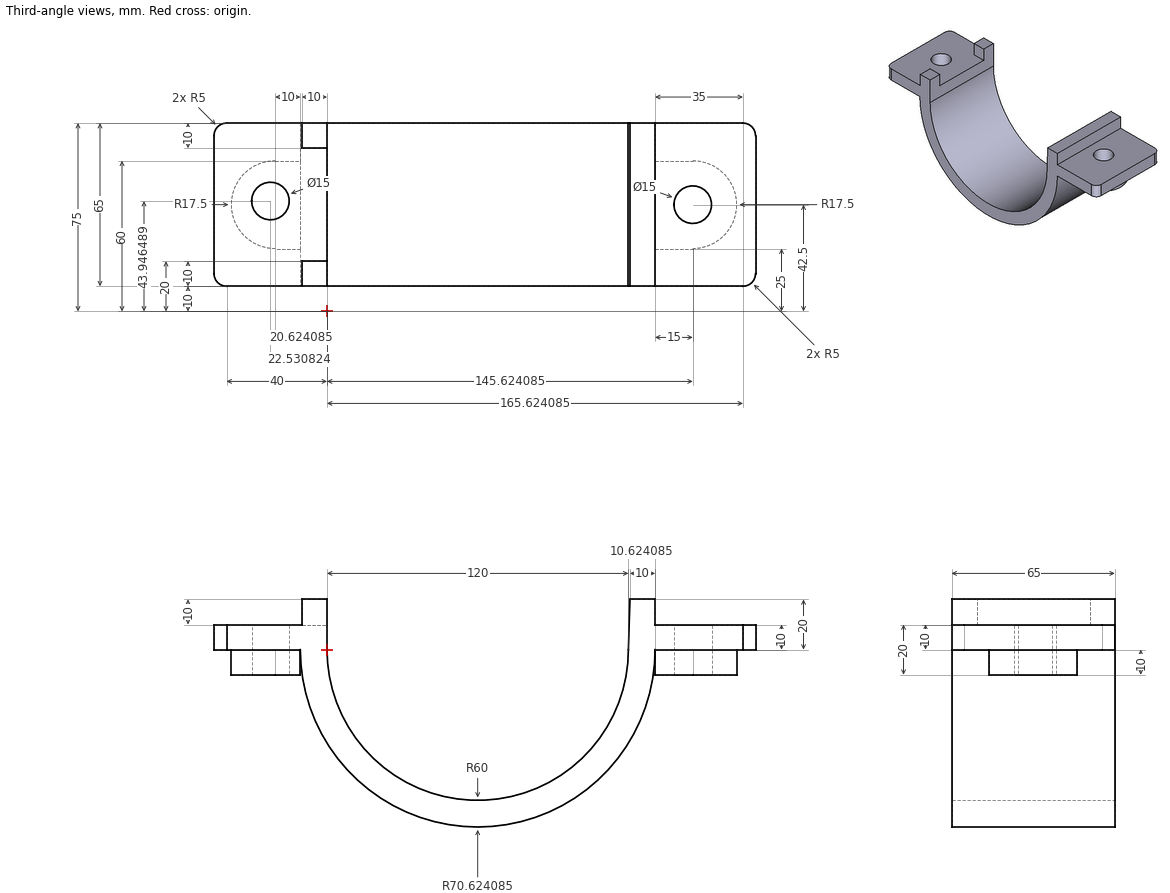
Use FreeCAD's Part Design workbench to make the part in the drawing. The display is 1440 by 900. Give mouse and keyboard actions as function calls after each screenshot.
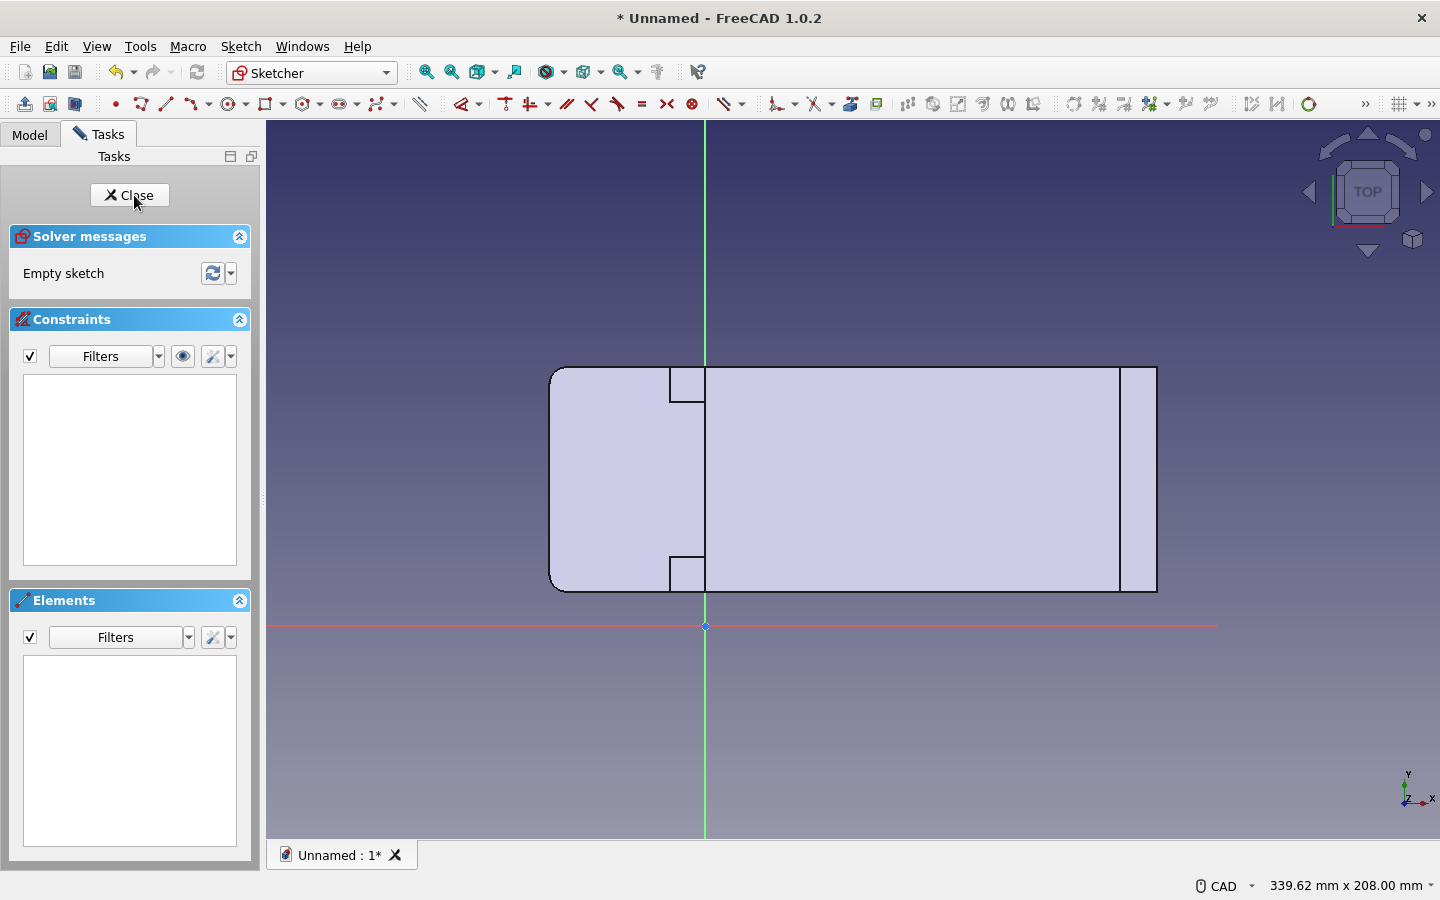
scroll(784, 480, down, 5)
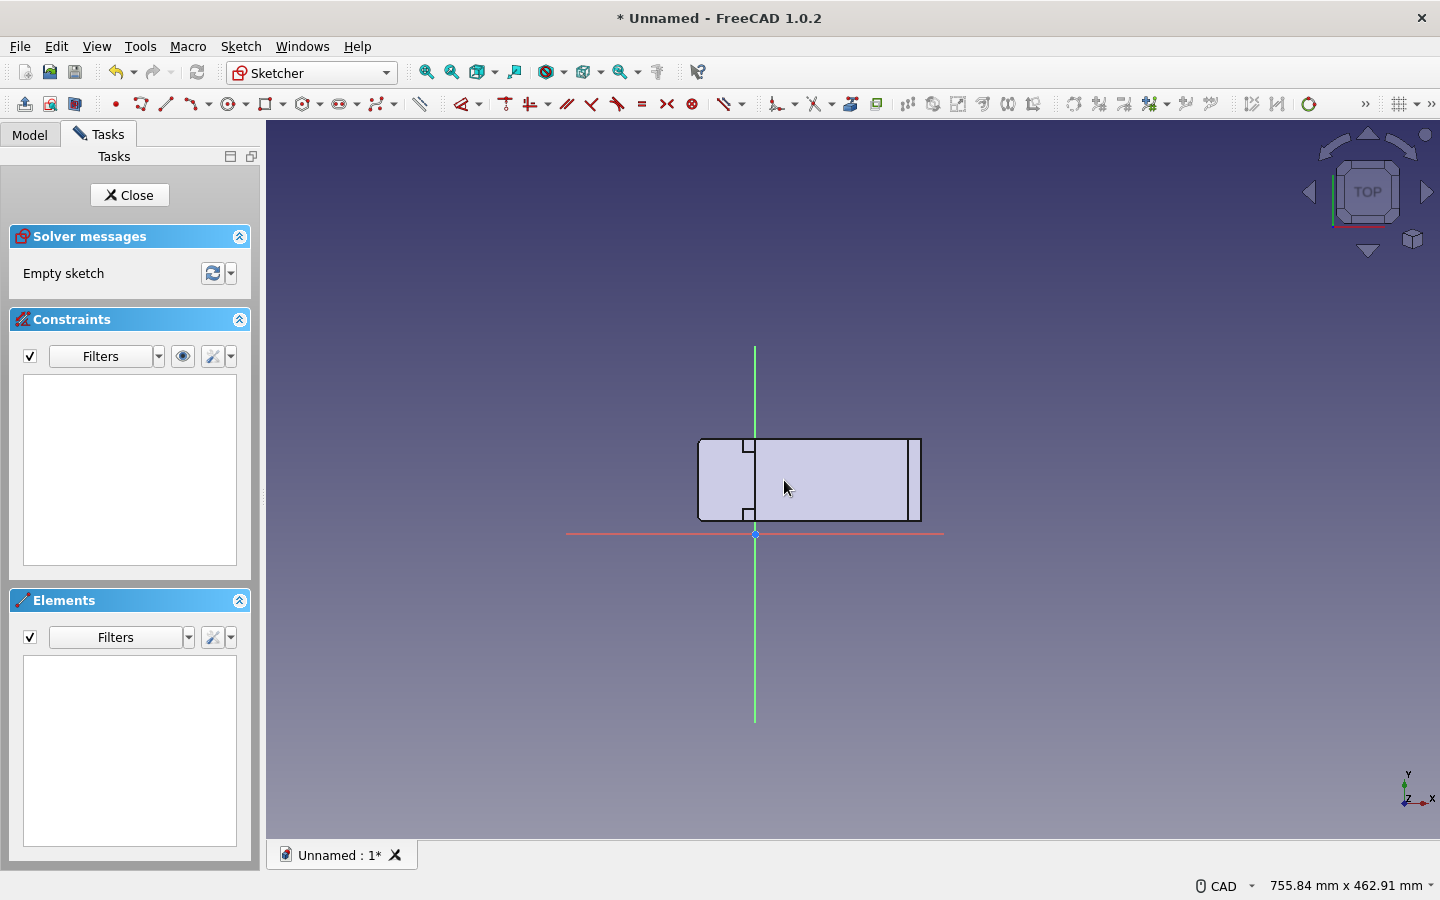
scroll(979, 480, up, 9)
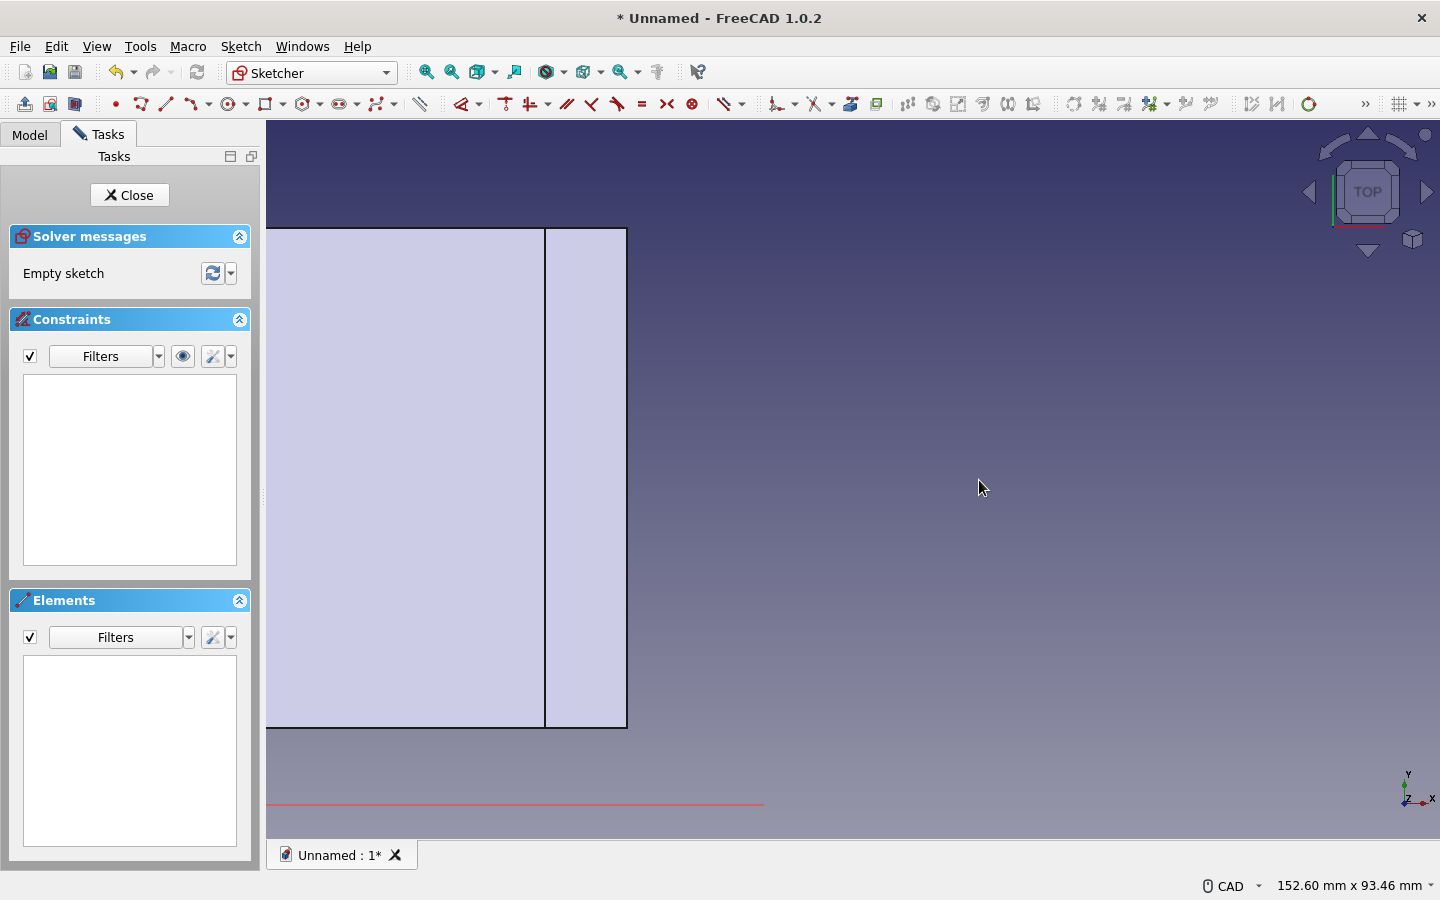
key(g)
key(m)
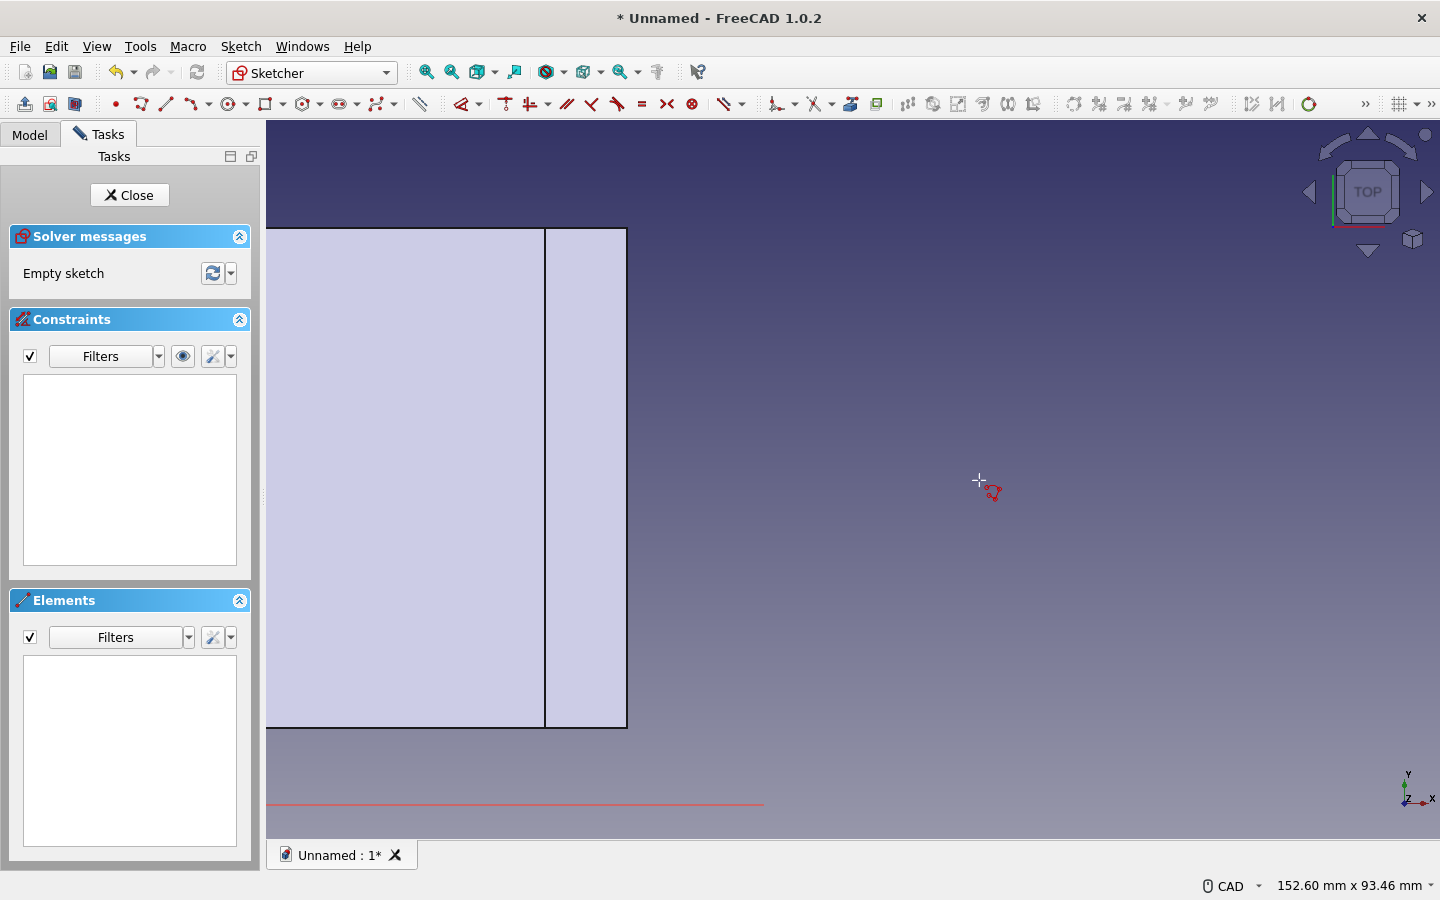
click(896, 228)
click(627, 228)
click(627, 728)
click(896, 728)
right_click(896, 728)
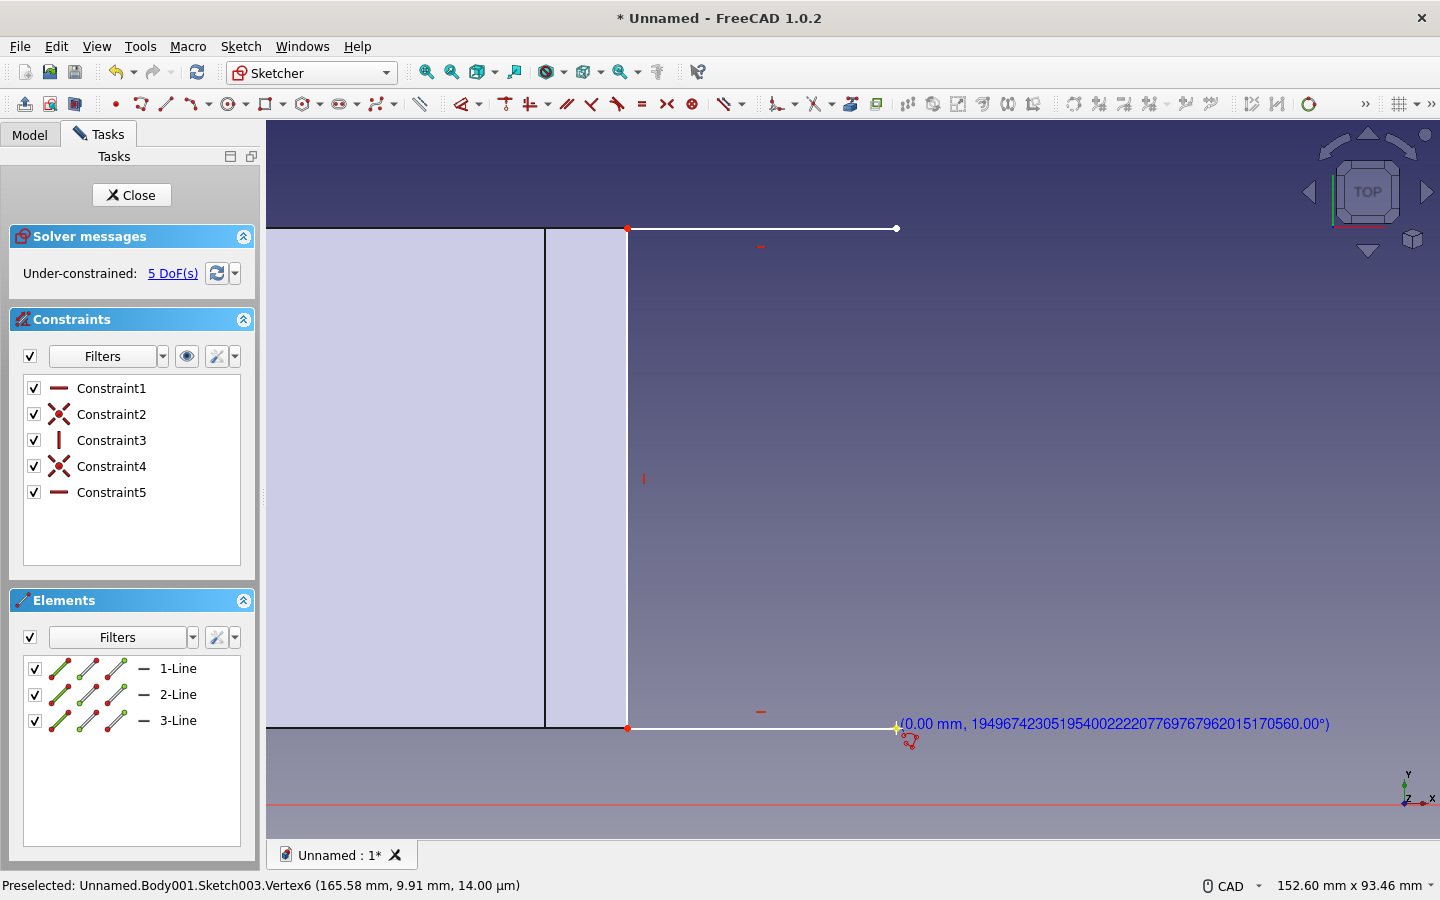
key(g)
key(l)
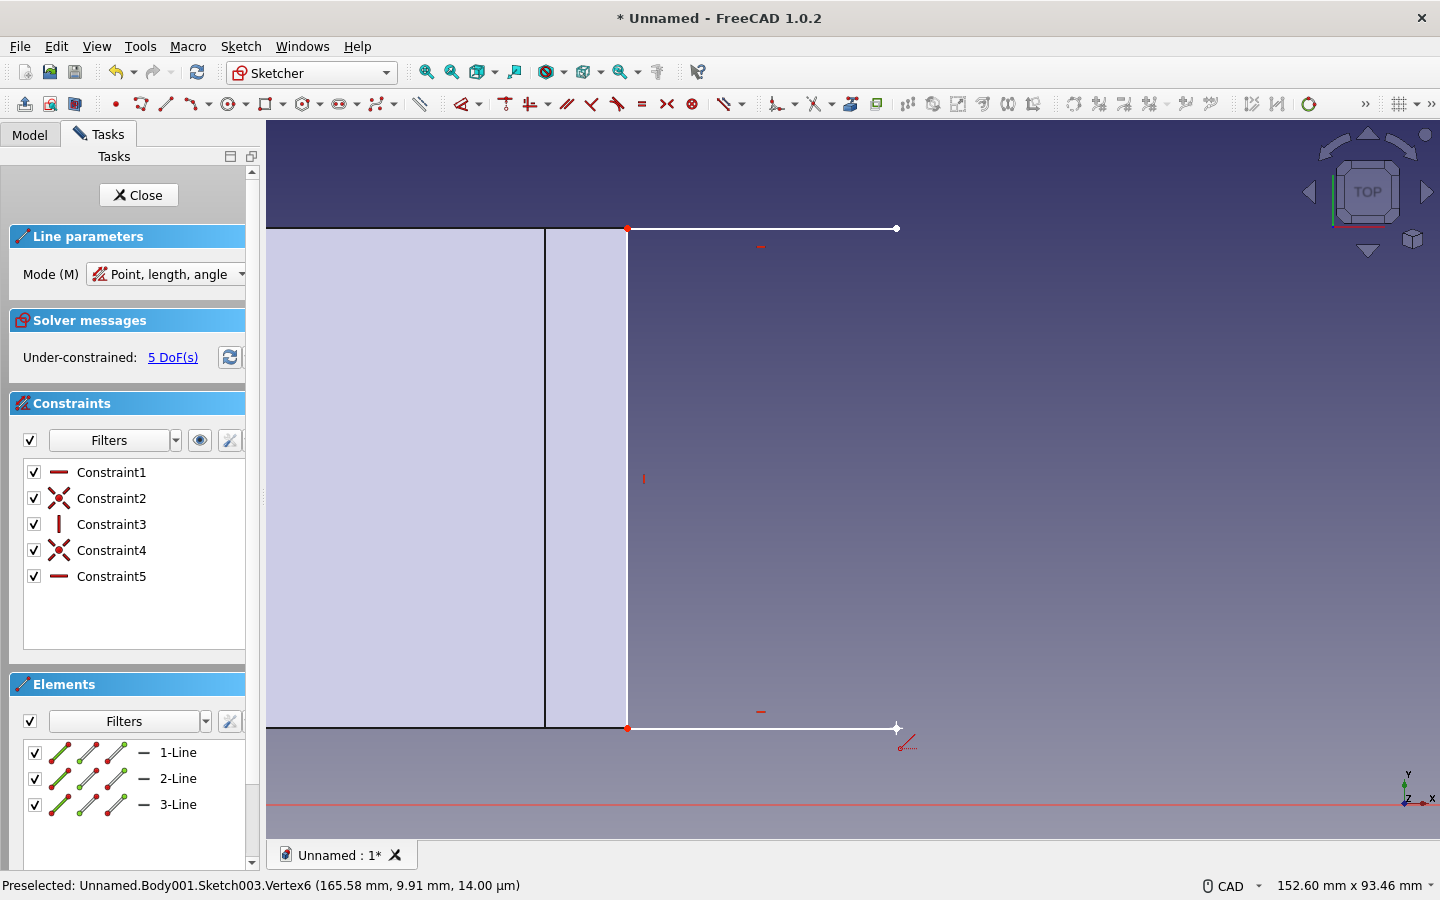
click(935, 690)
click(935, 267)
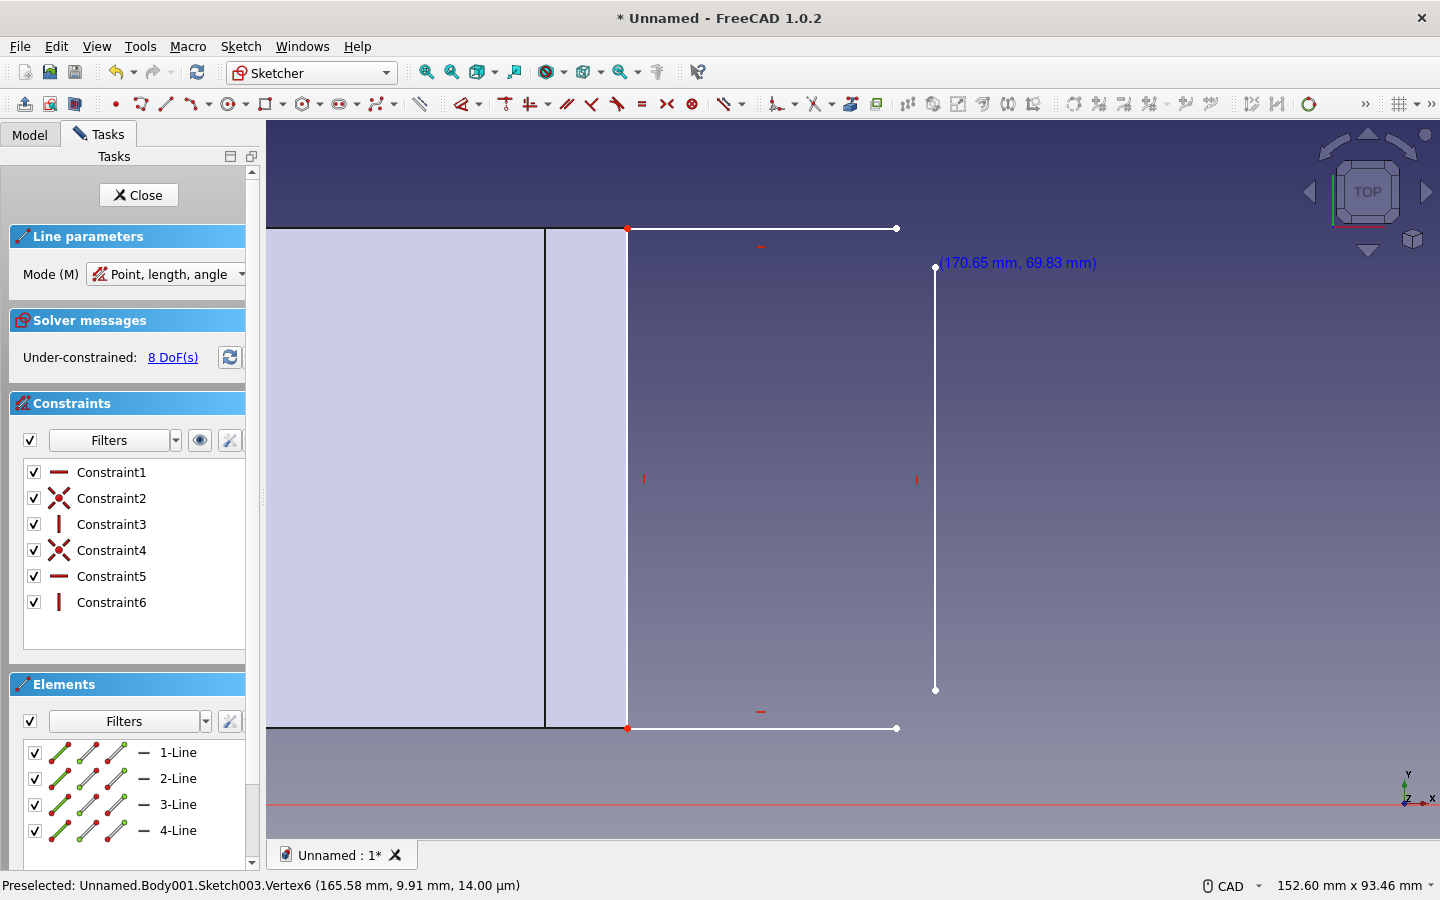
key(g)
key(3)
key(a)